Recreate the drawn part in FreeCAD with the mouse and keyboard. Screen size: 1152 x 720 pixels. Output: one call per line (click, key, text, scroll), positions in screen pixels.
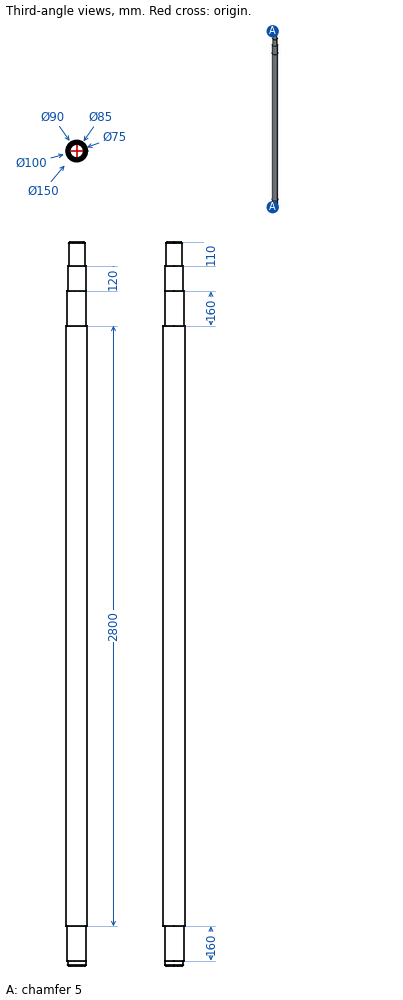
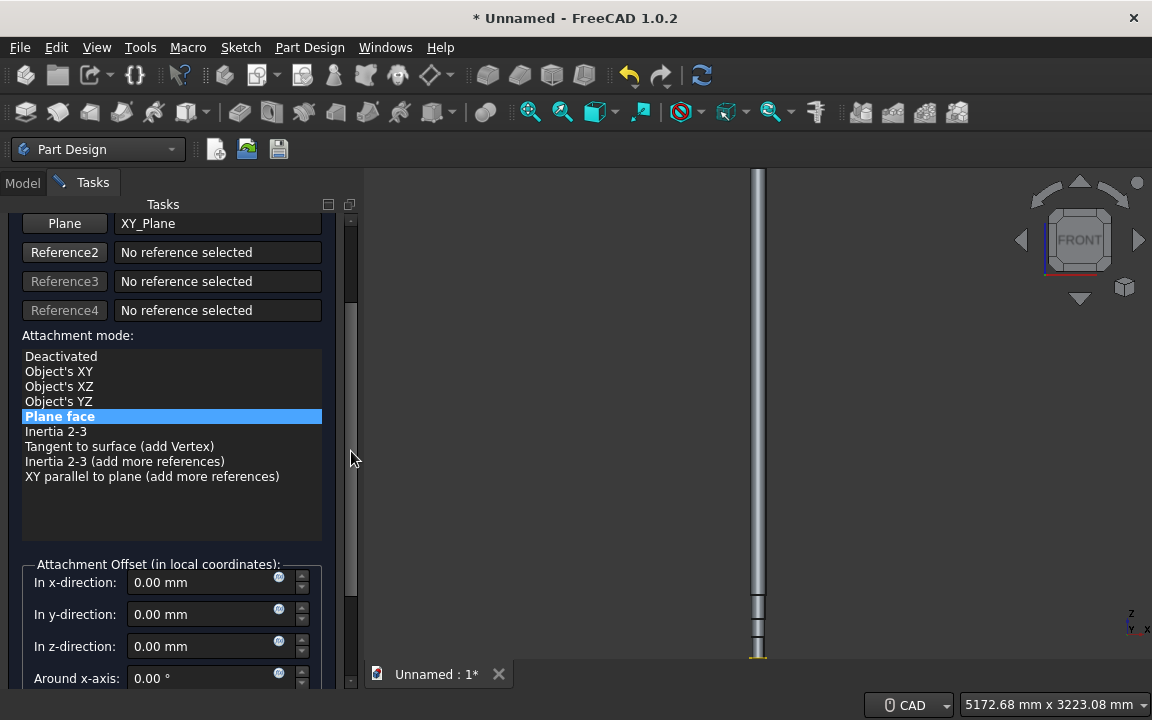
triple_click(210, 586)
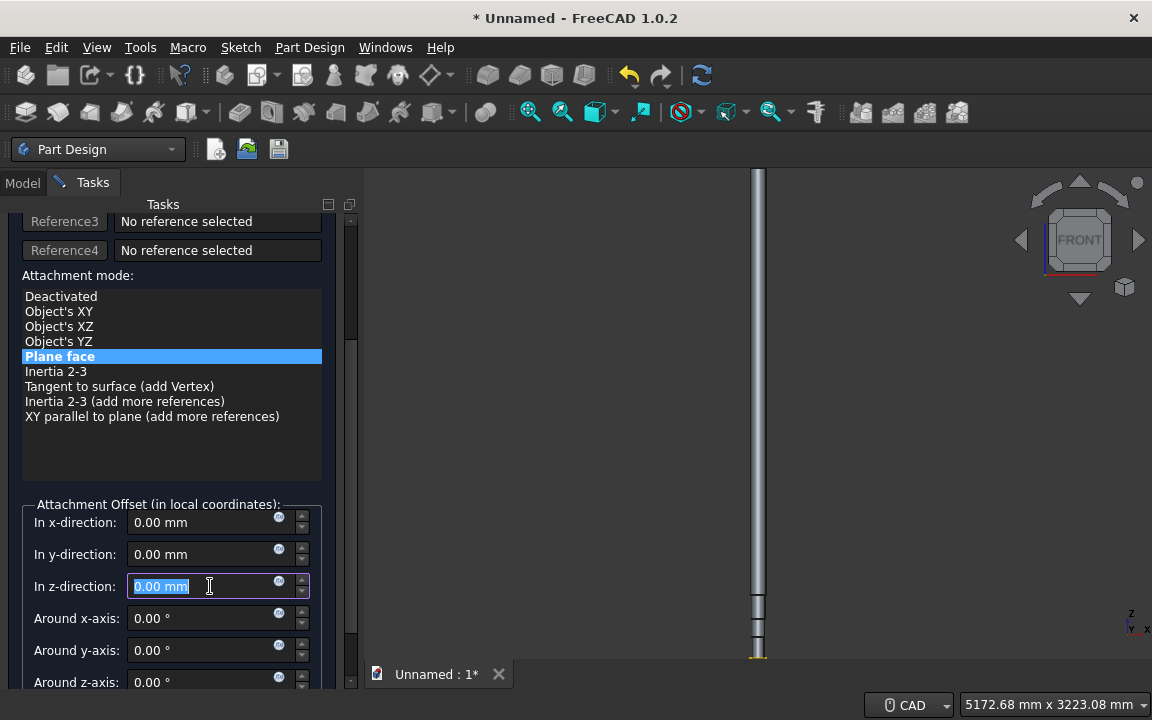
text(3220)
key(Tab)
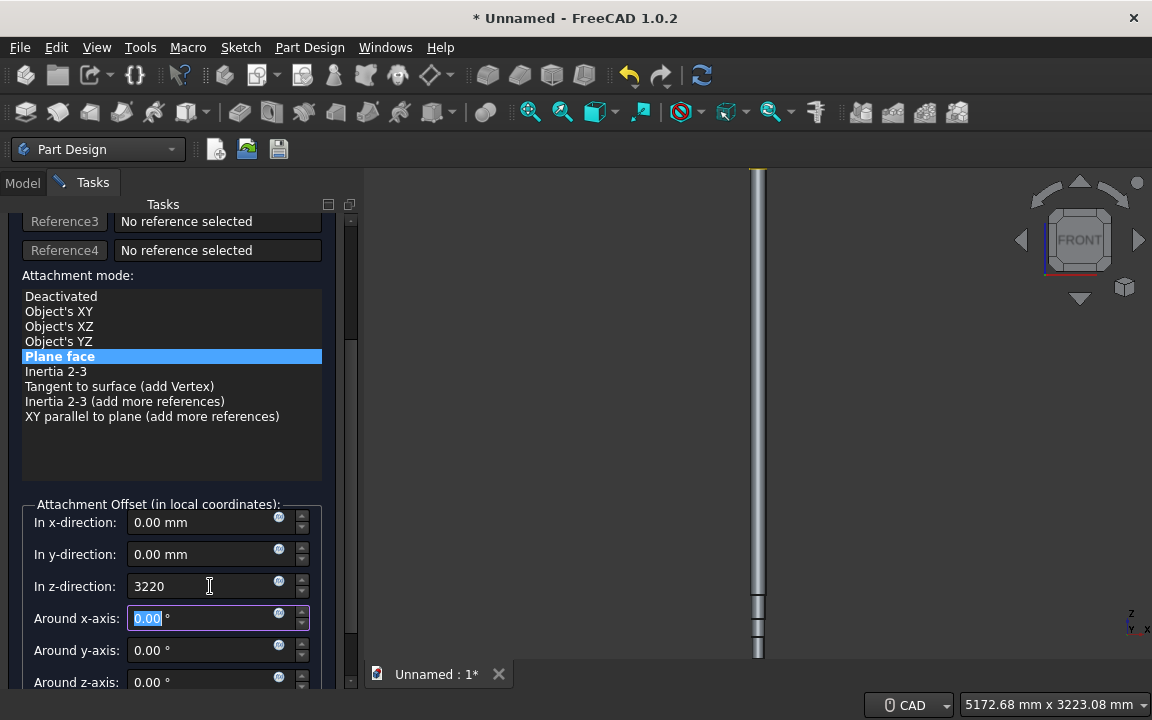
scroll(351, 451, up, 4)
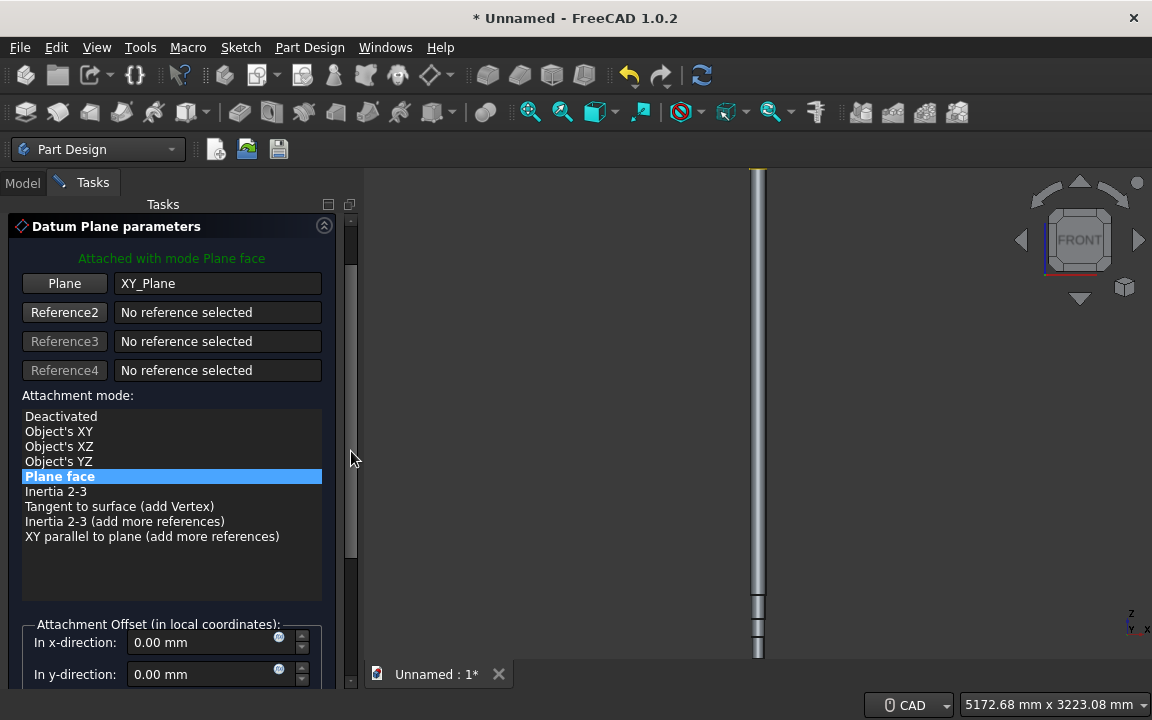
click(124, 243)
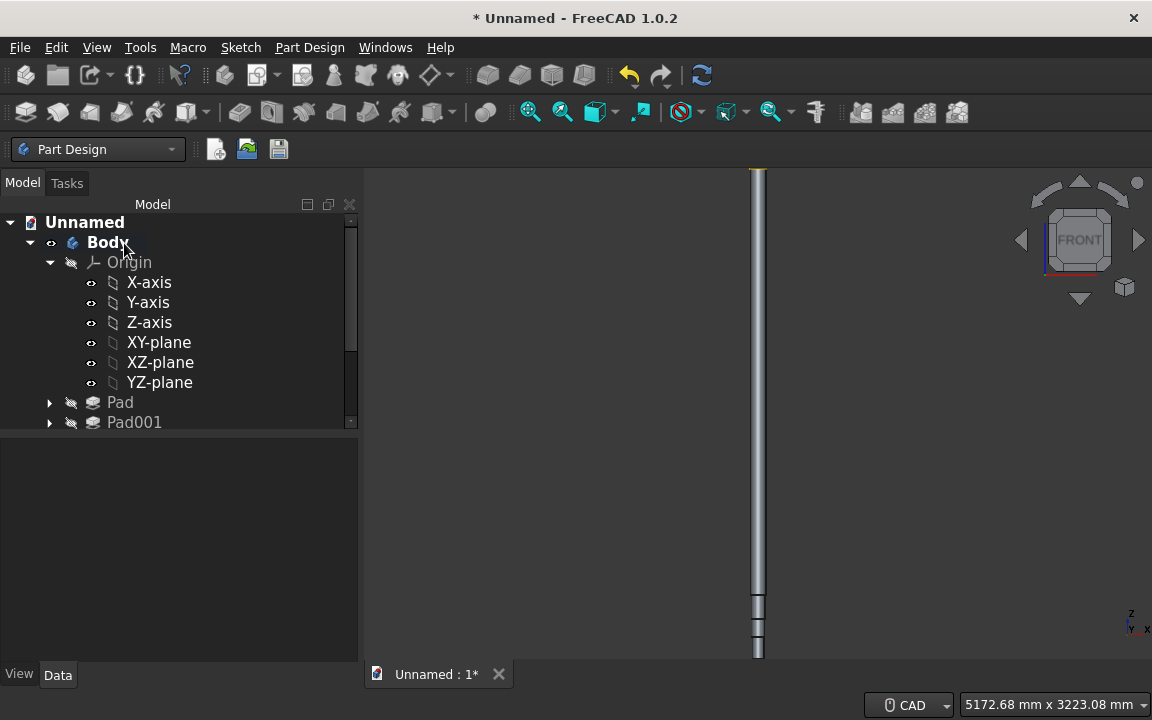
scroll(100, 318, down, 3)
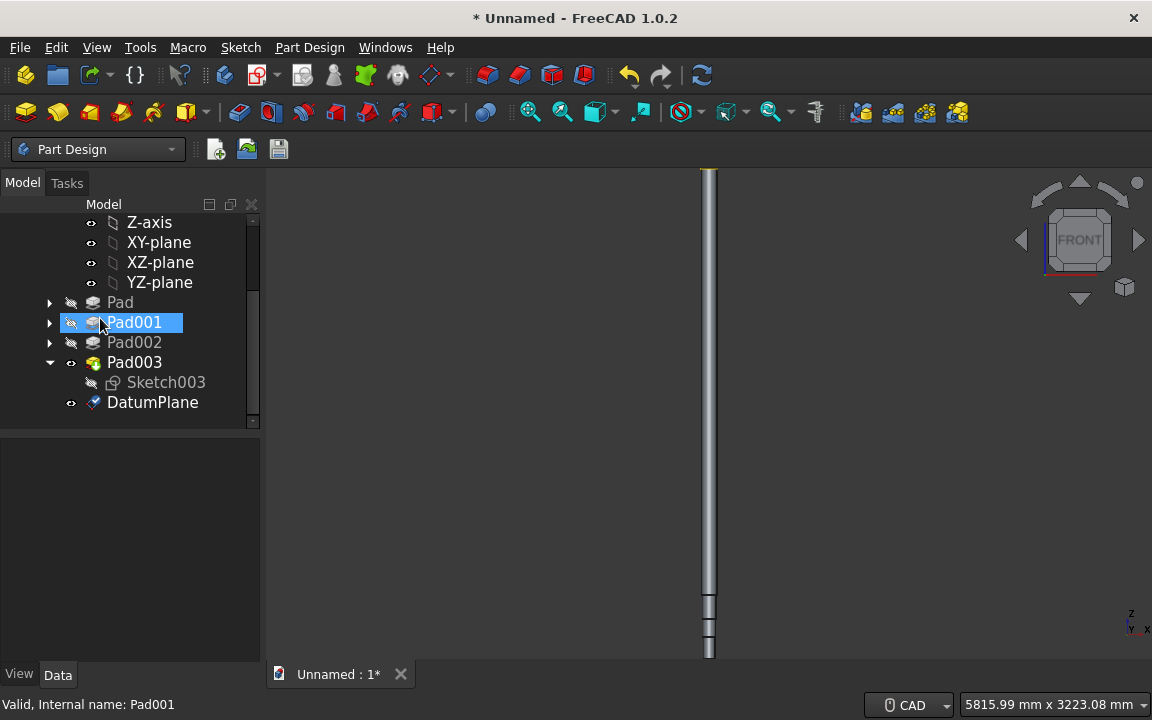
click(116, 403)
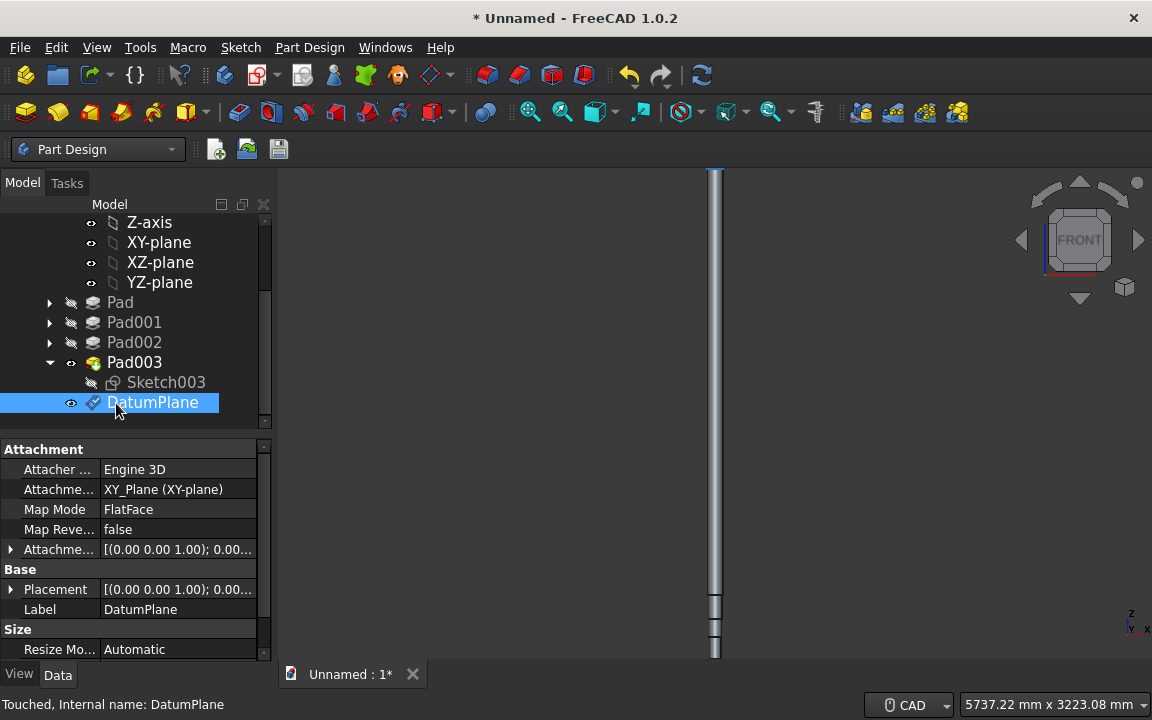
click(258, 76)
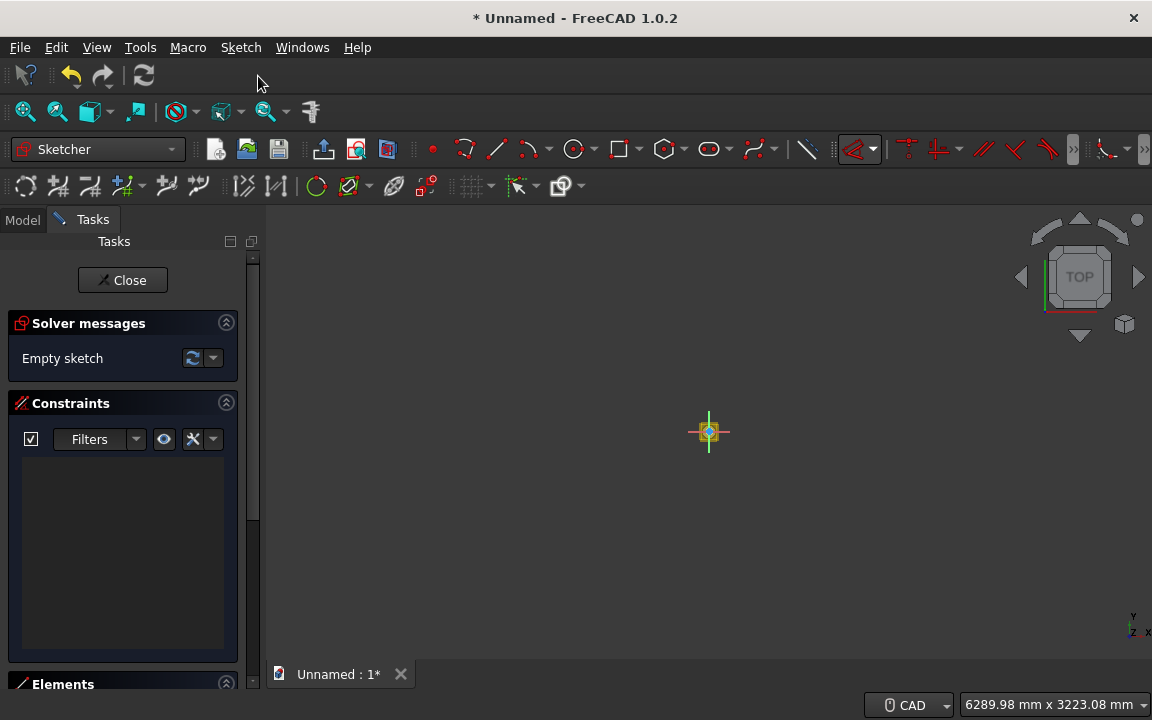
scroll(713, 432, up, 15)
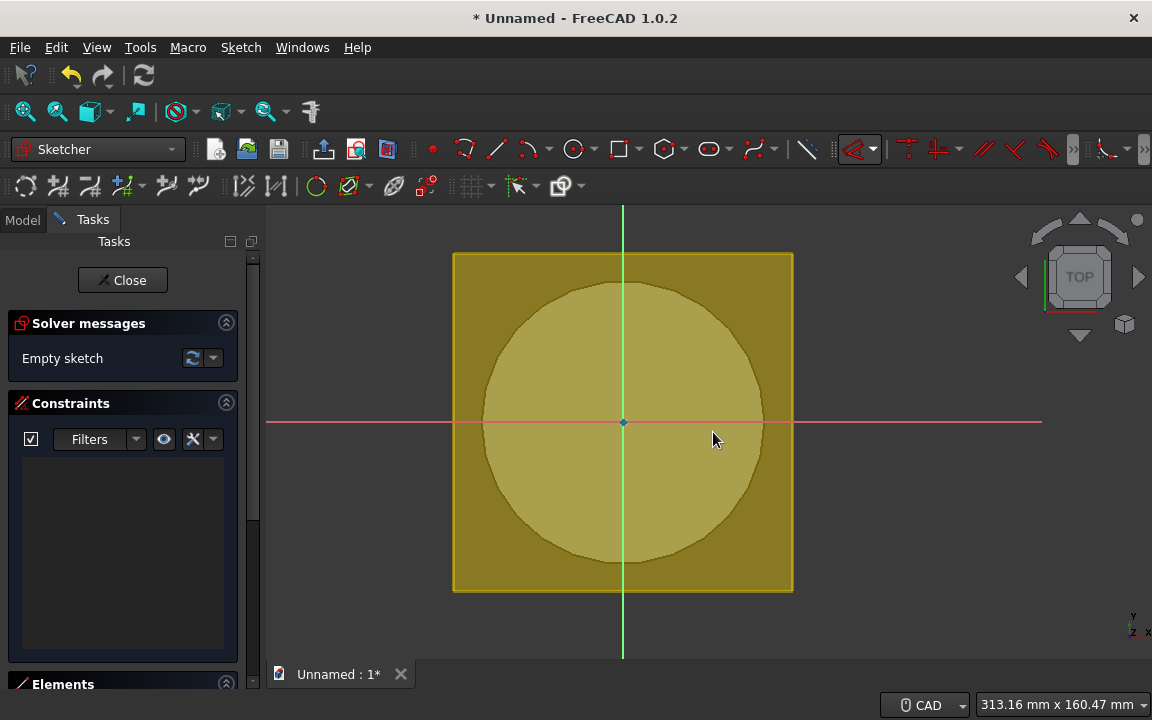
click(574, 150)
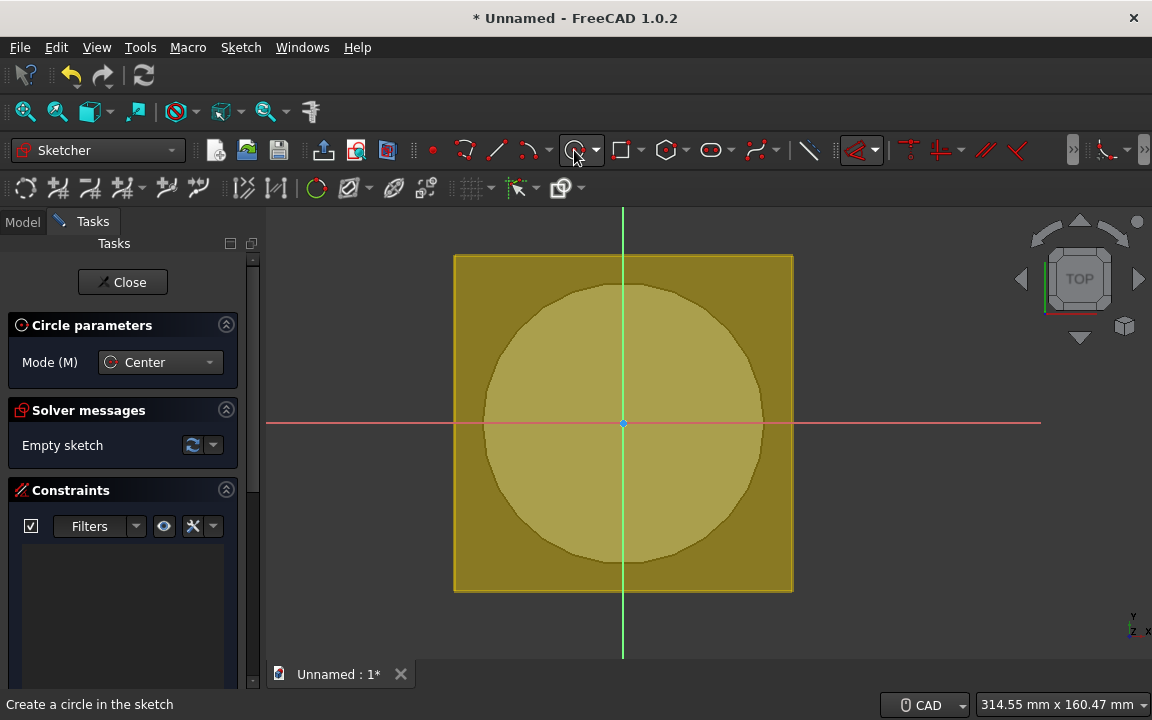
click(623, 423)
click(713, 334)
key(Escape)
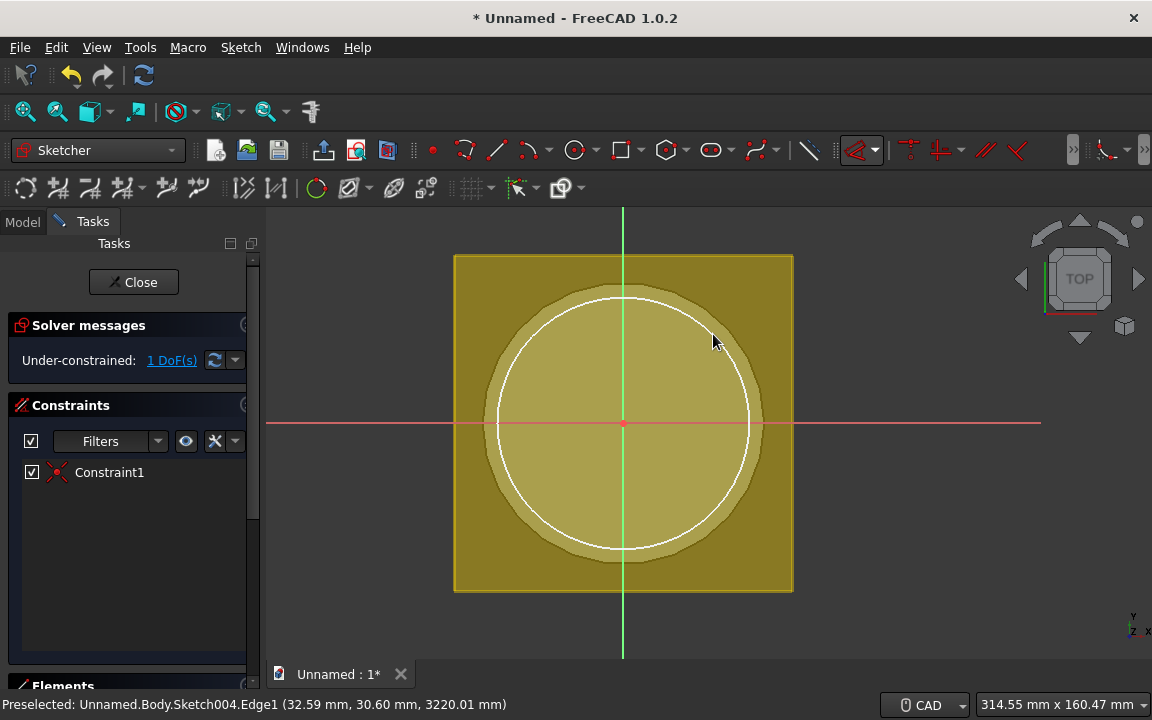
click(712, 334)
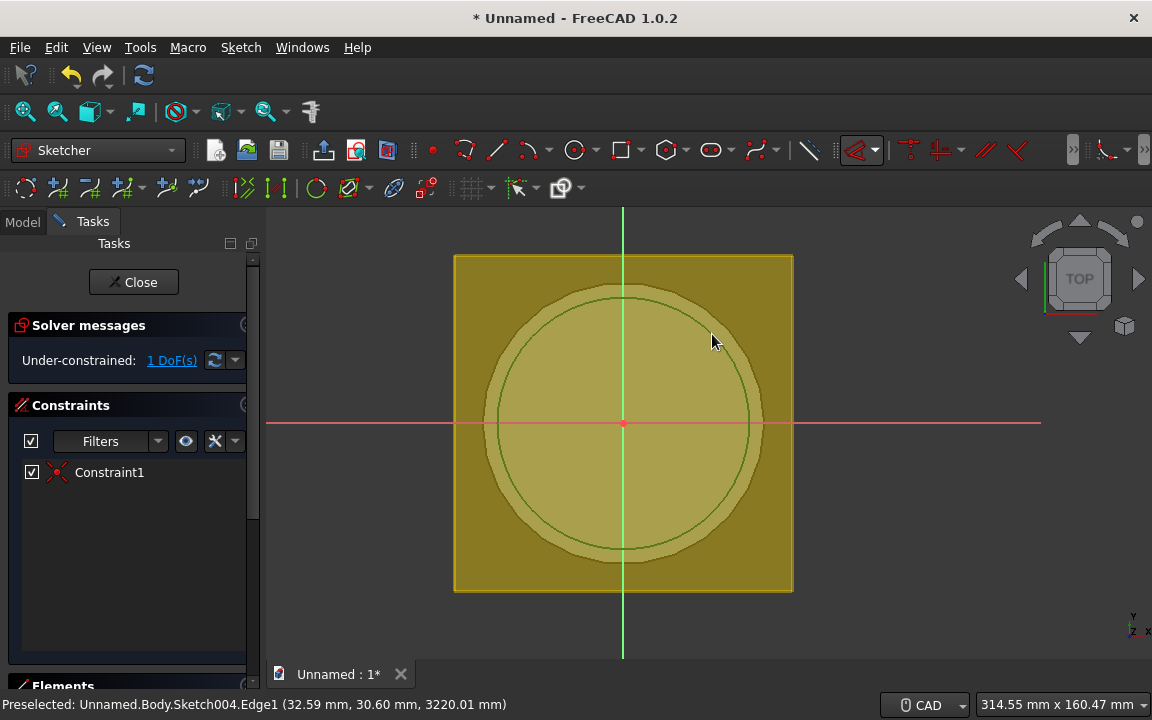
click(878, 150)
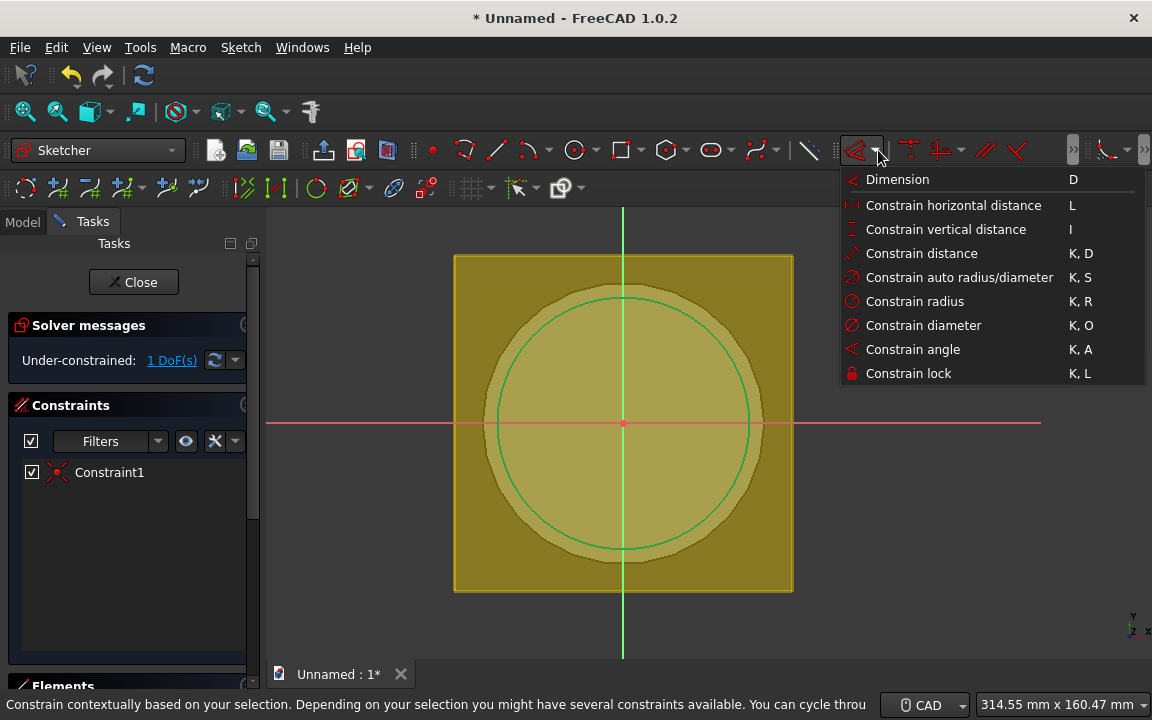
click(993, 325)